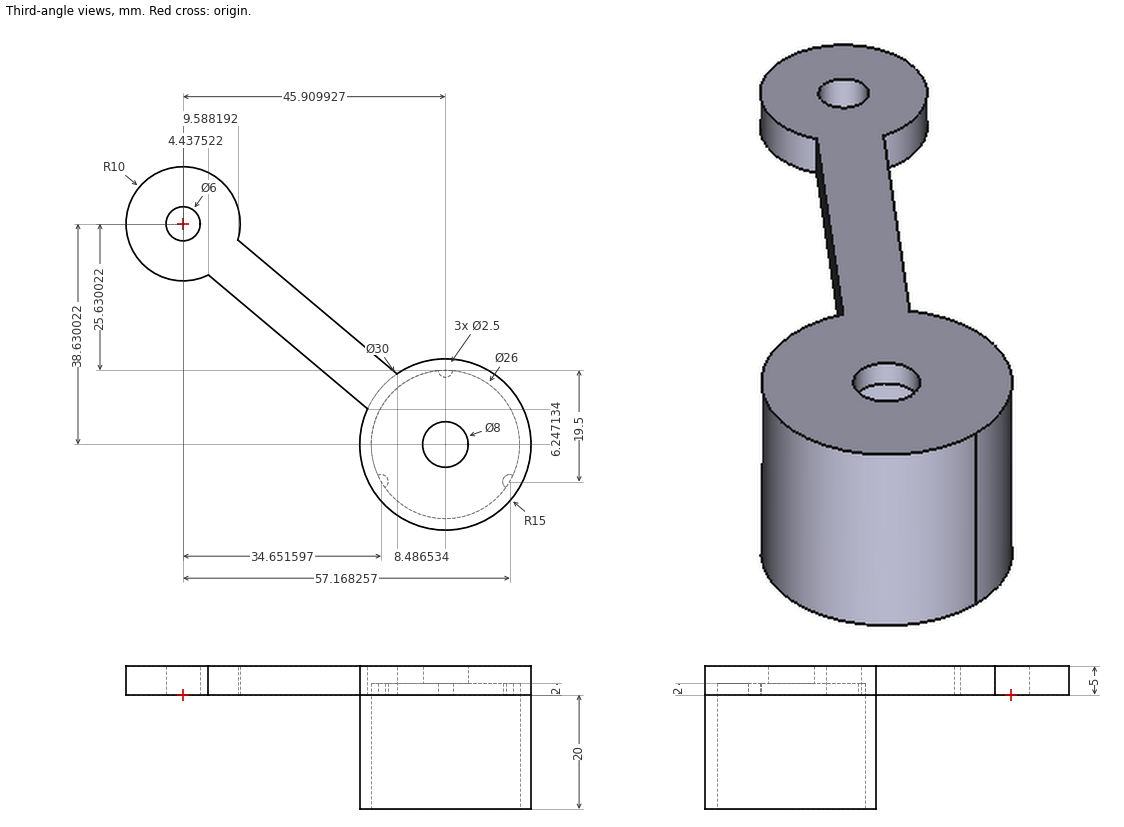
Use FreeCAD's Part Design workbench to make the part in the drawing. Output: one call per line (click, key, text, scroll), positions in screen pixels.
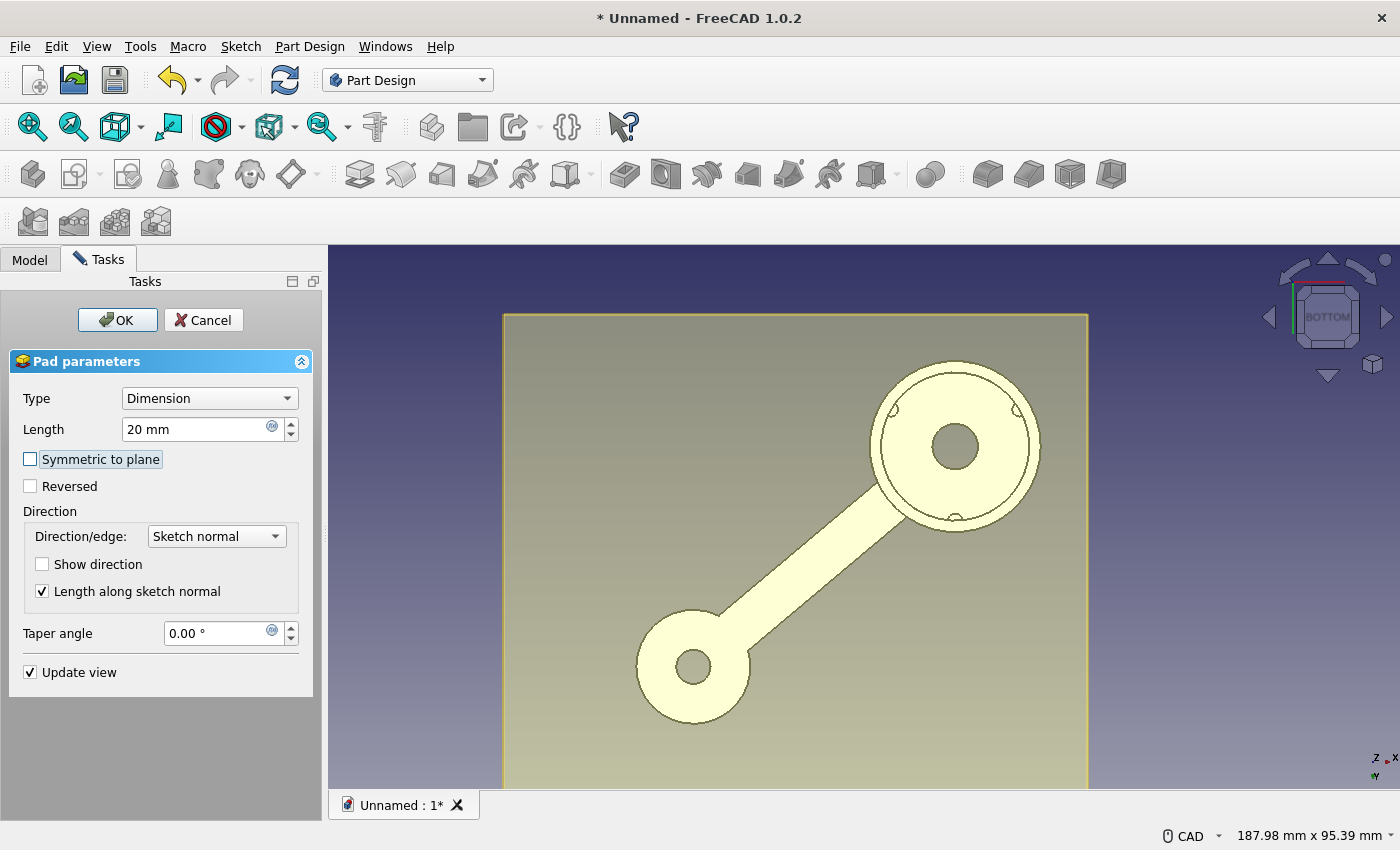
click(118, 320)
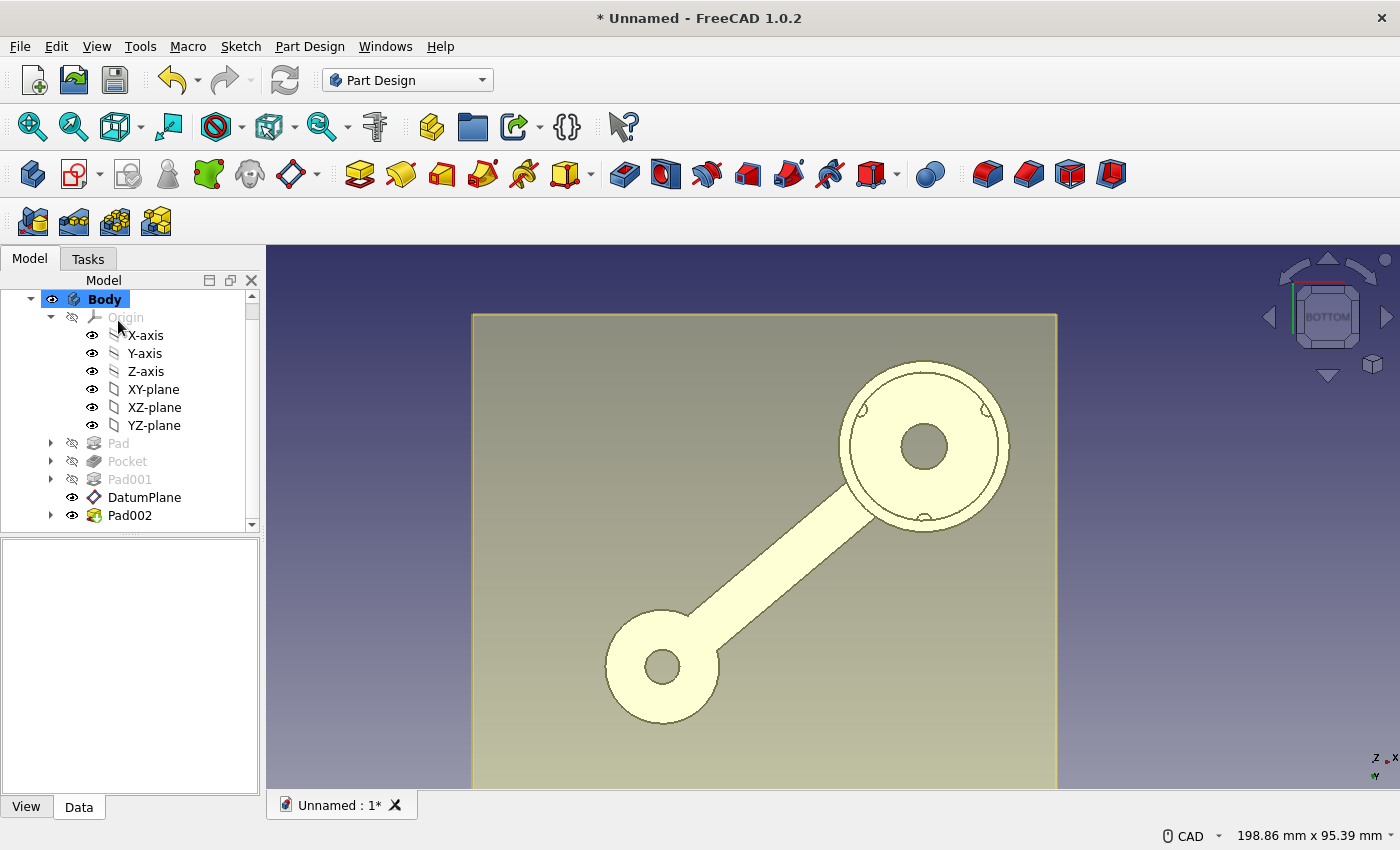
click(117, 497)
key(space)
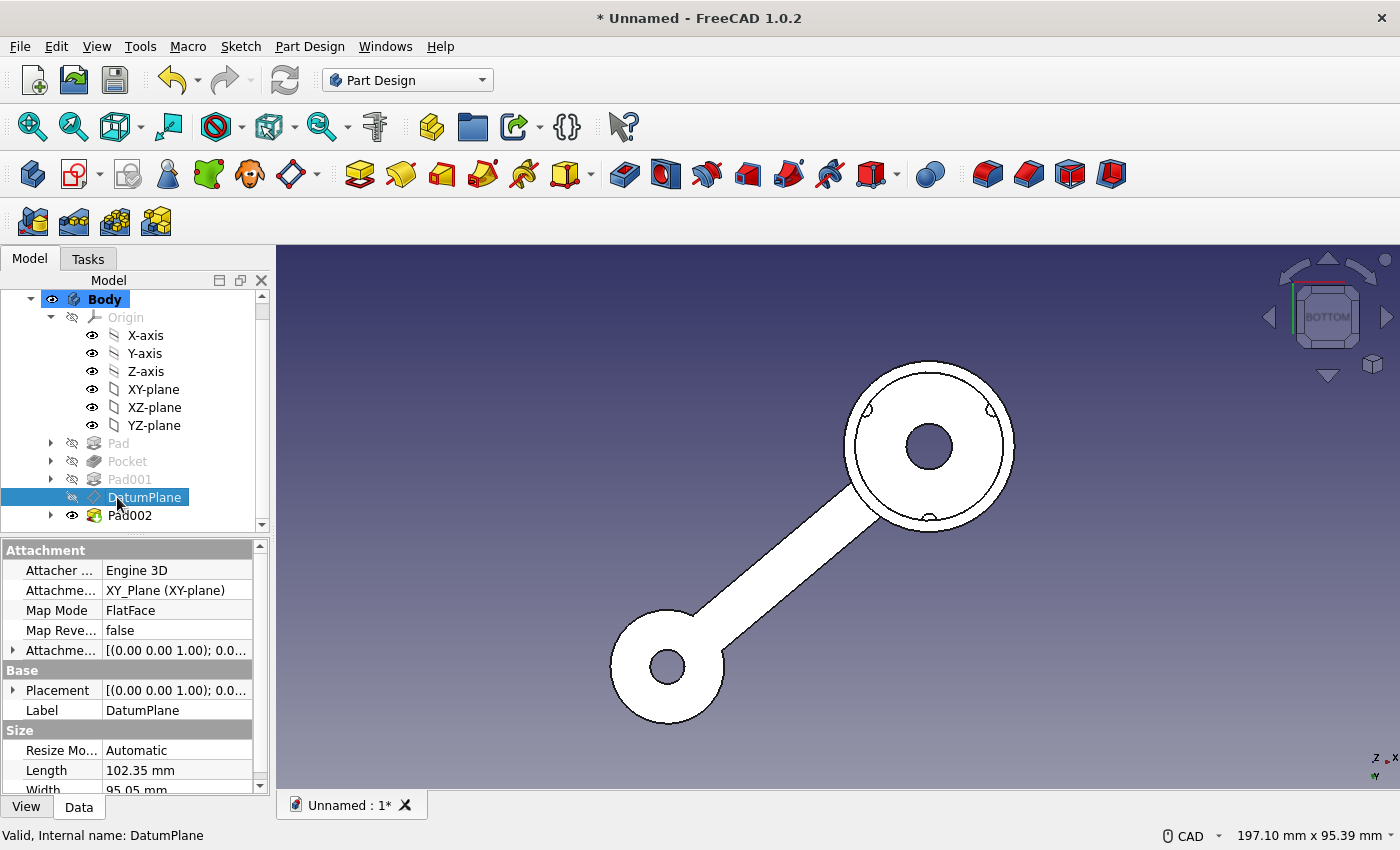
key(0)